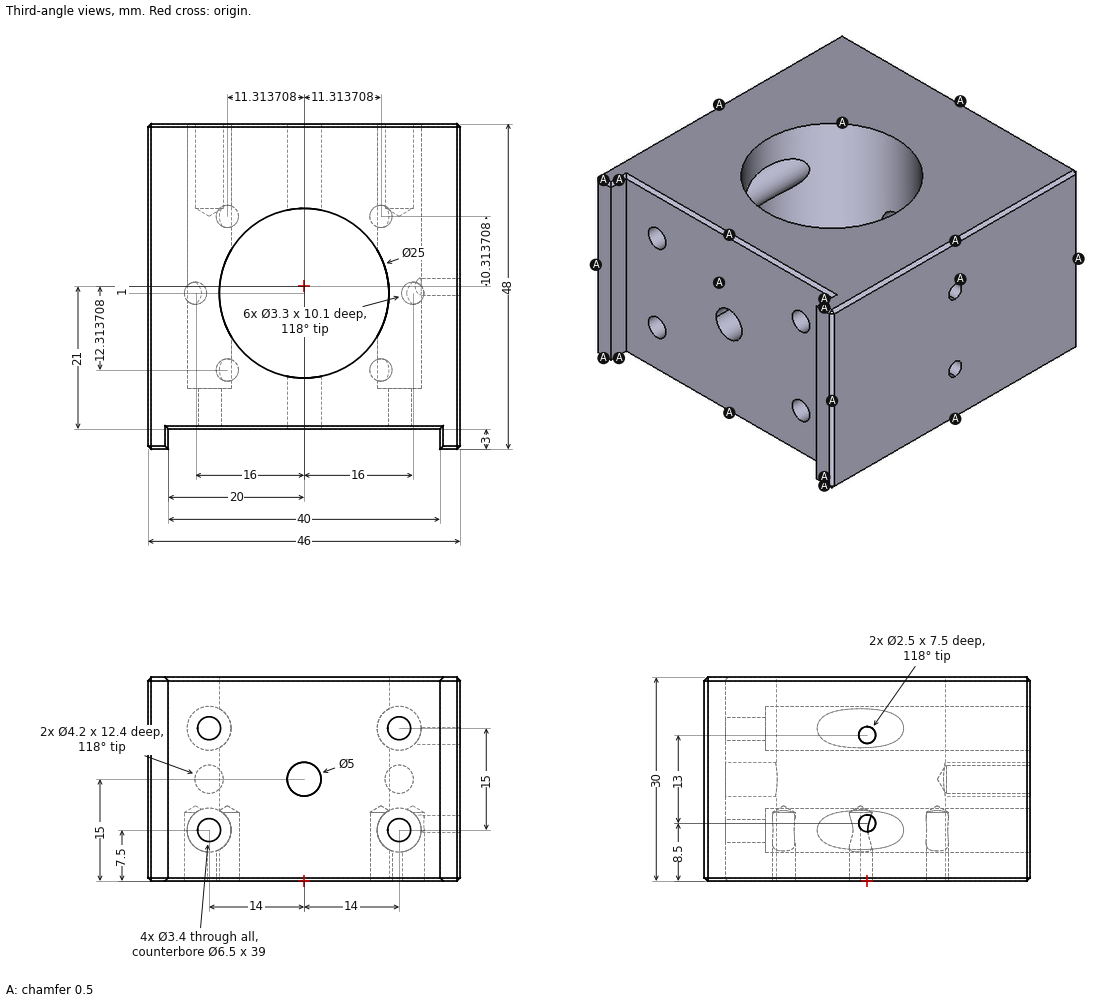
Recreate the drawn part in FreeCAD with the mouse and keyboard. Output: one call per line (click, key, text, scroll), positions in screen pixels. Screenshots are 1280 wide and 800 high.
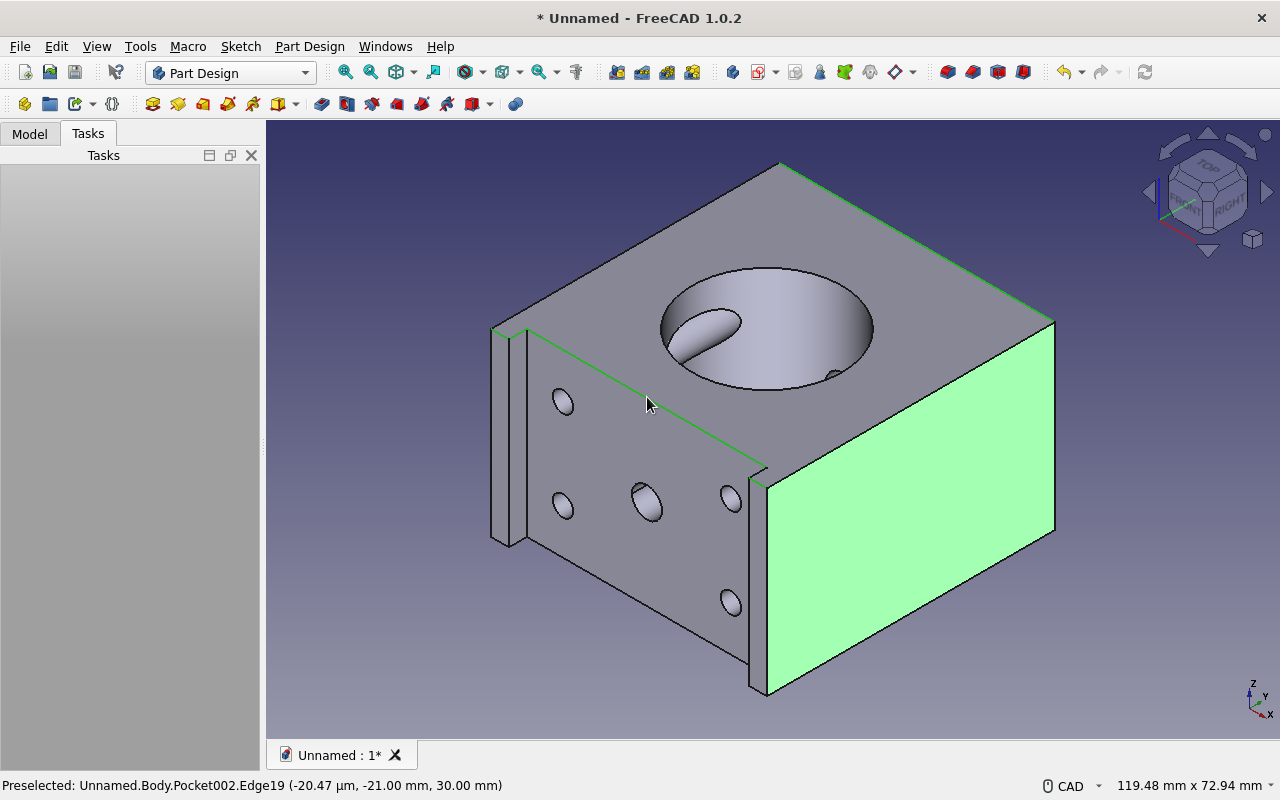
key(2)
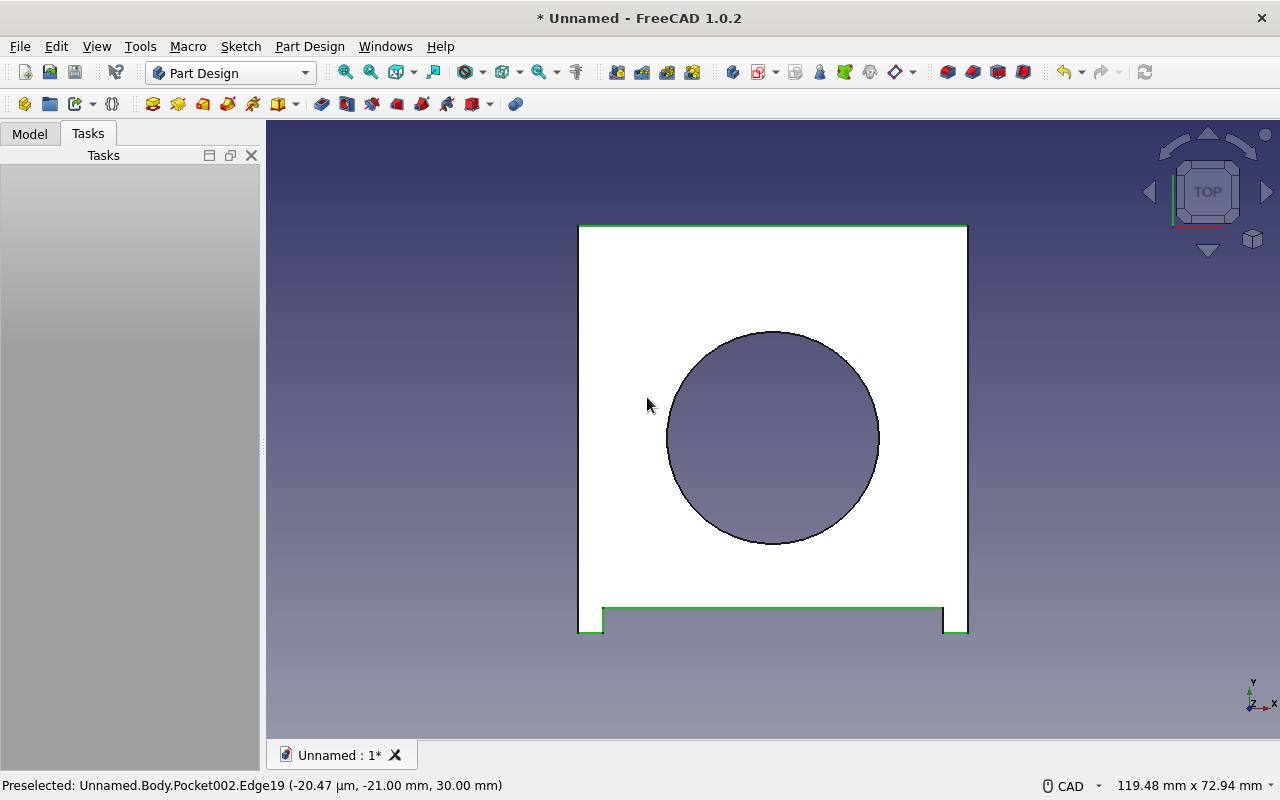
click(943, 619, ctrl)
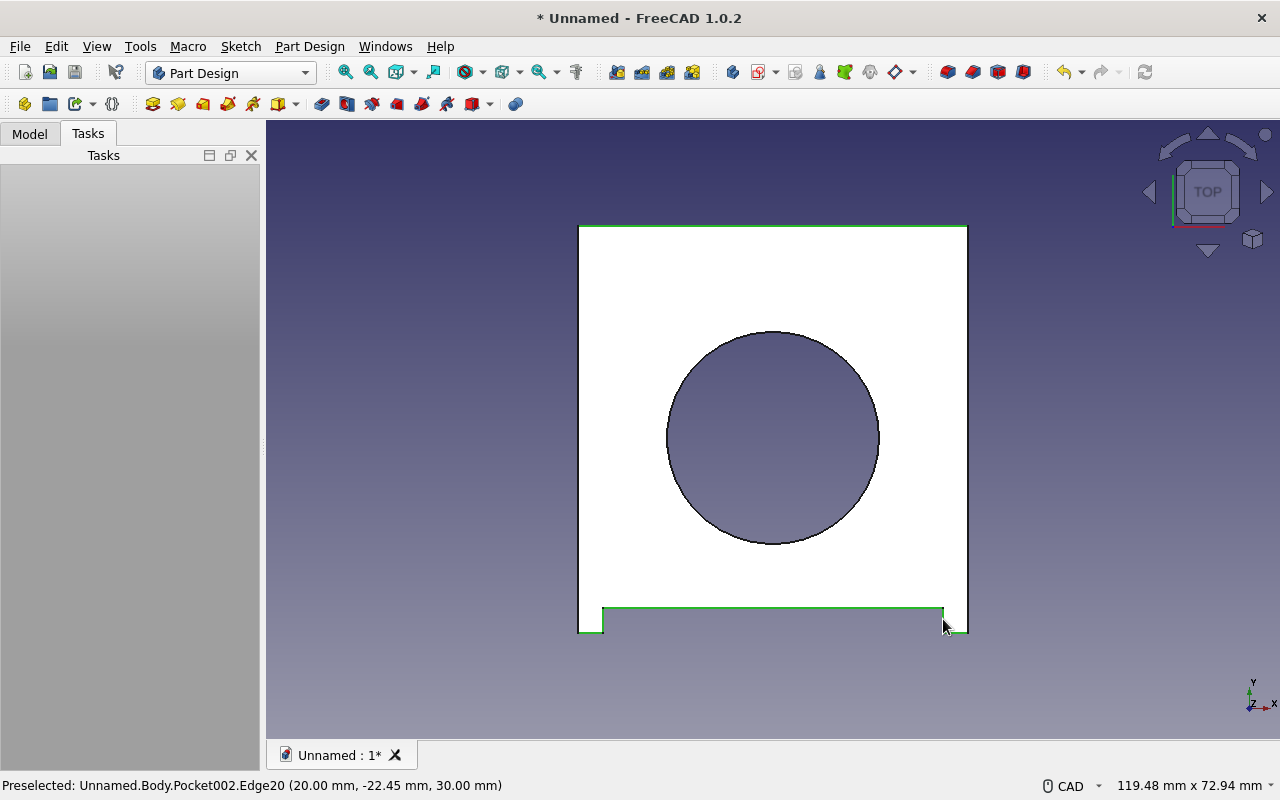
key(1)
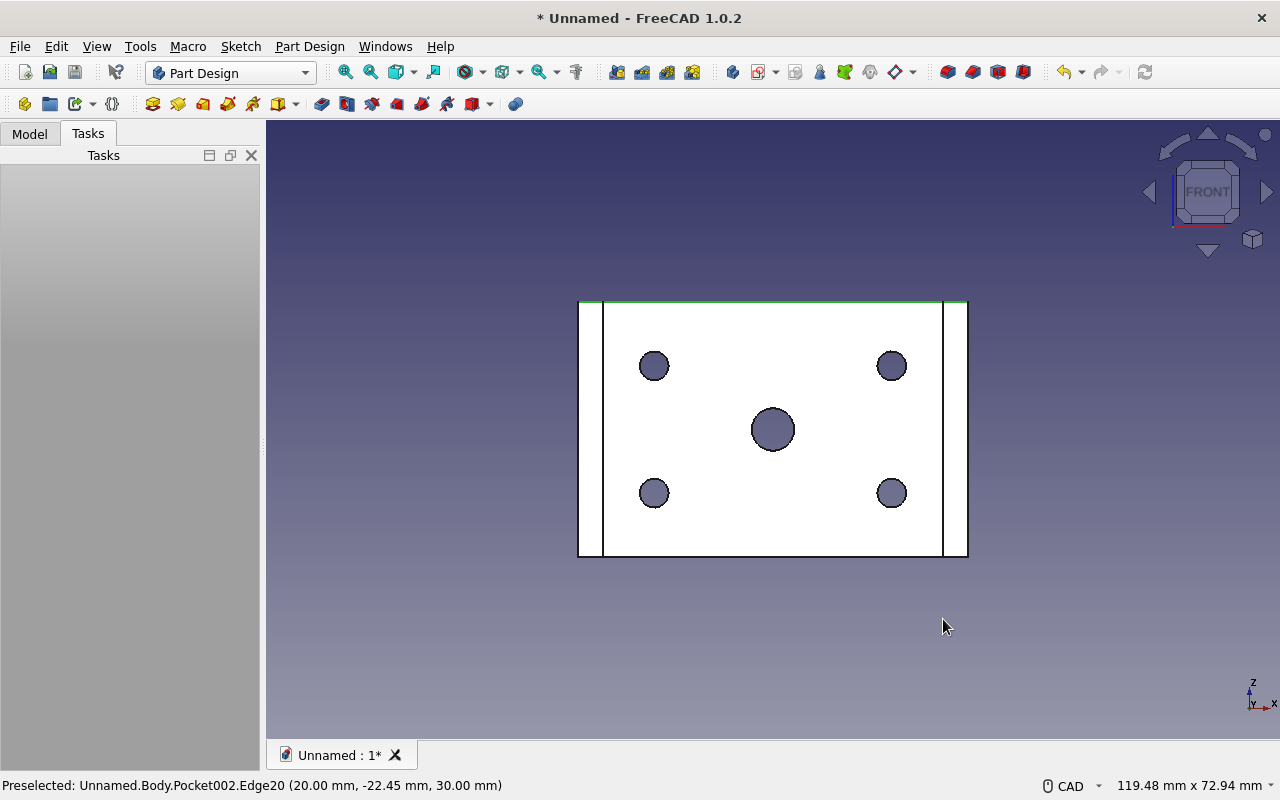
click(346, 72)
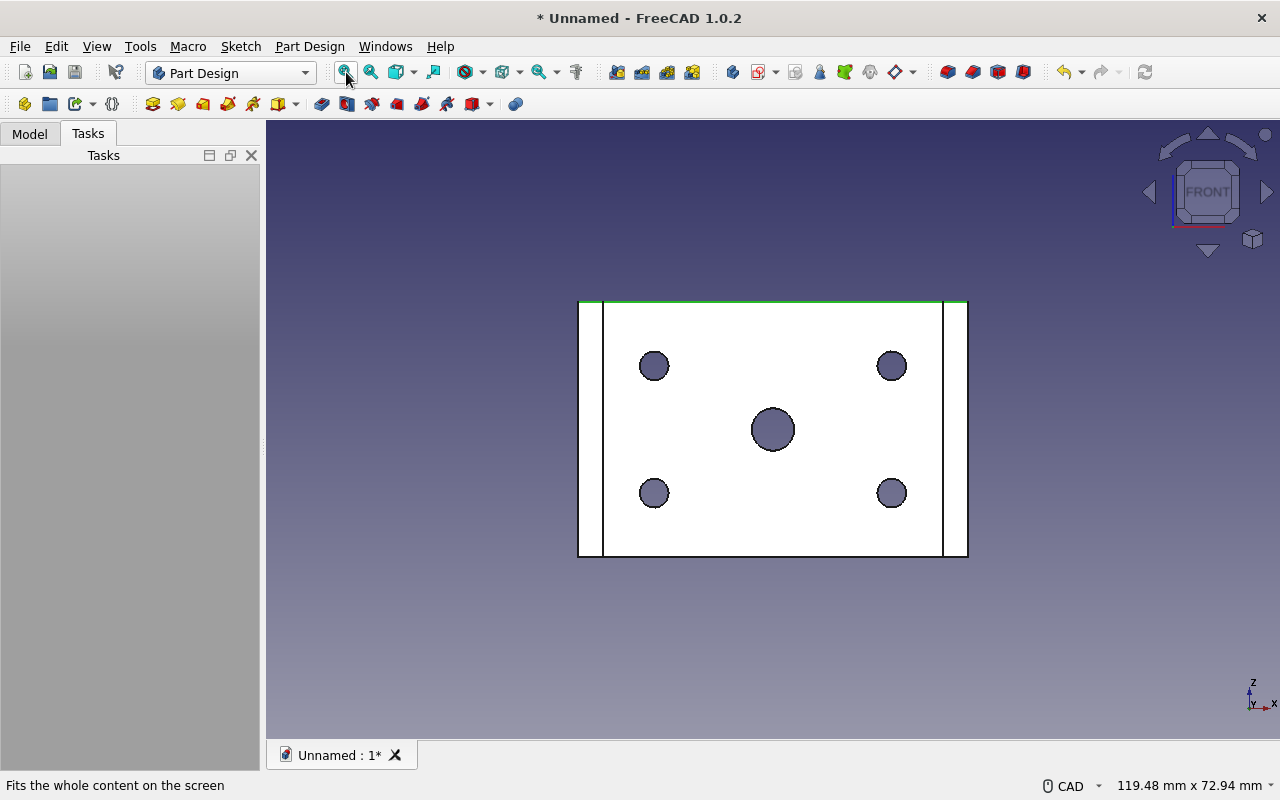
click(955, 556, ctrl)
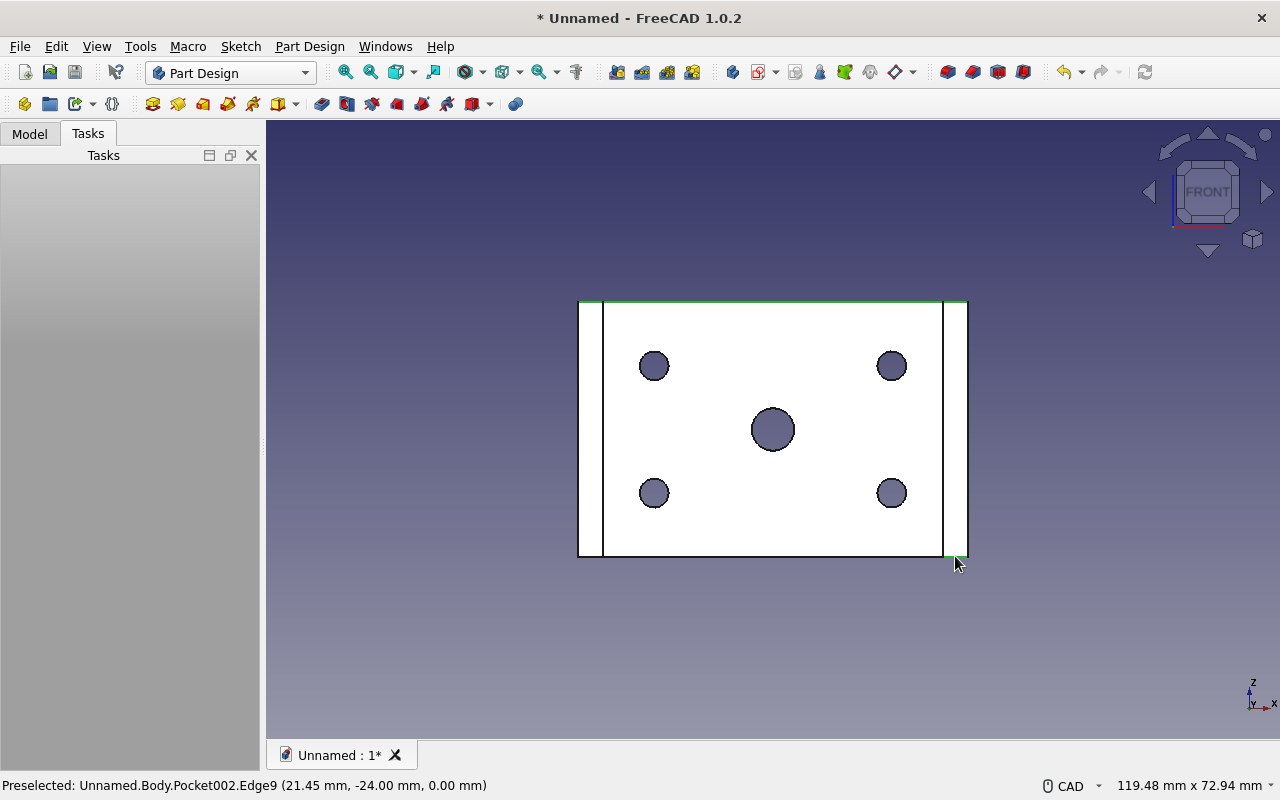
click(773, 556, ctrl)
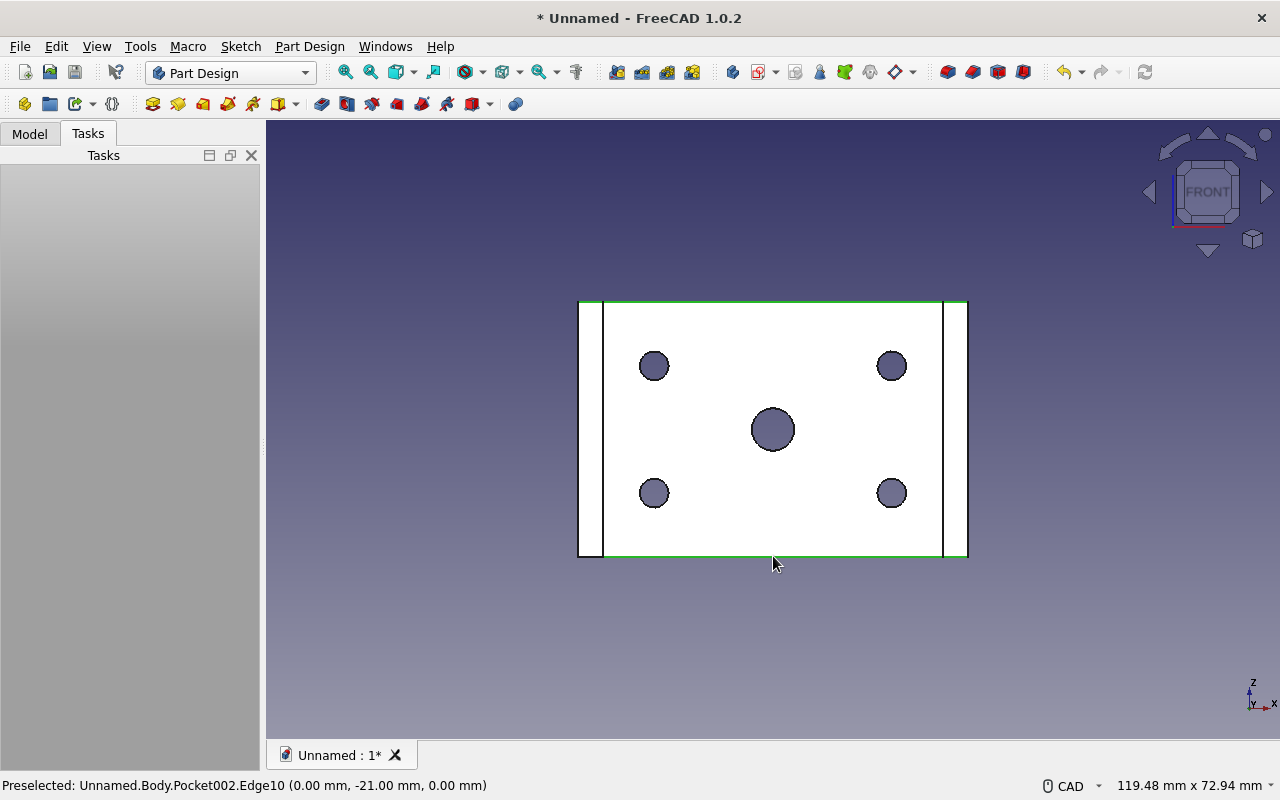
click(591, 556, ctrl)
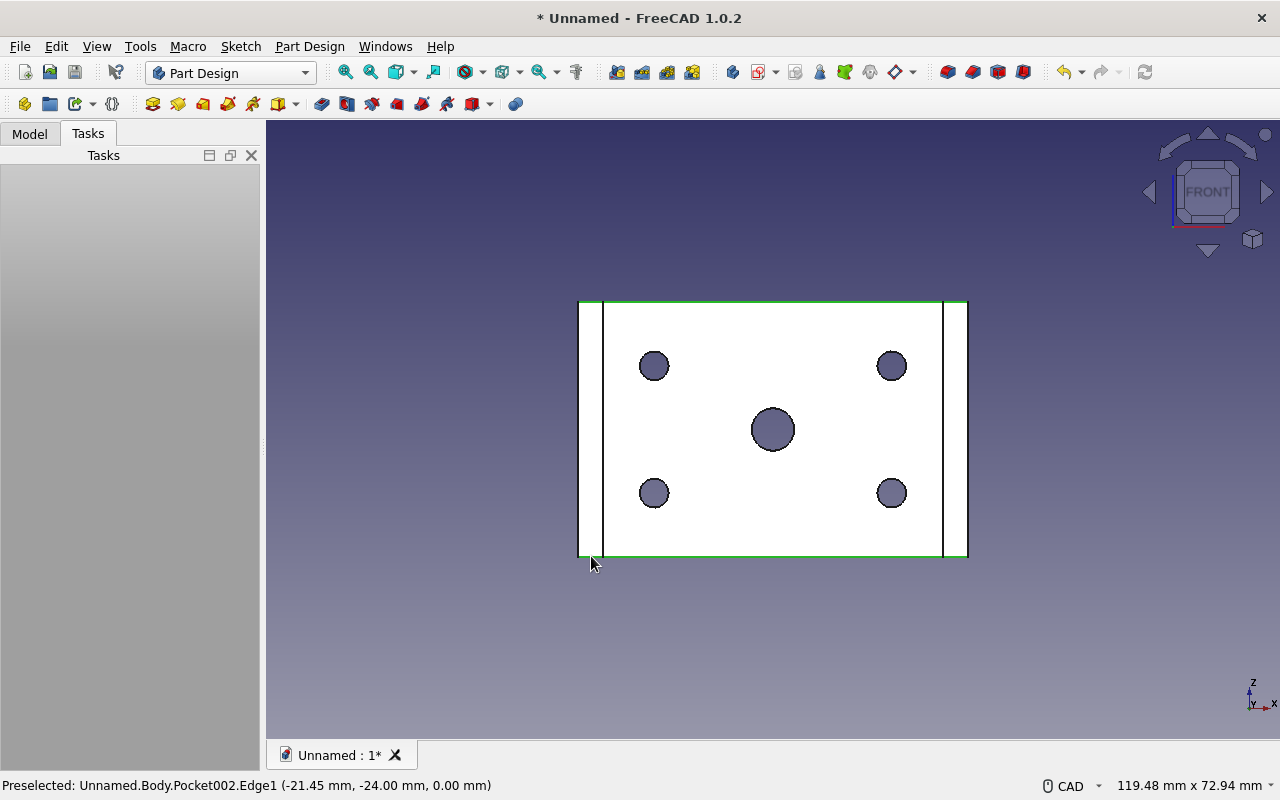
key(3)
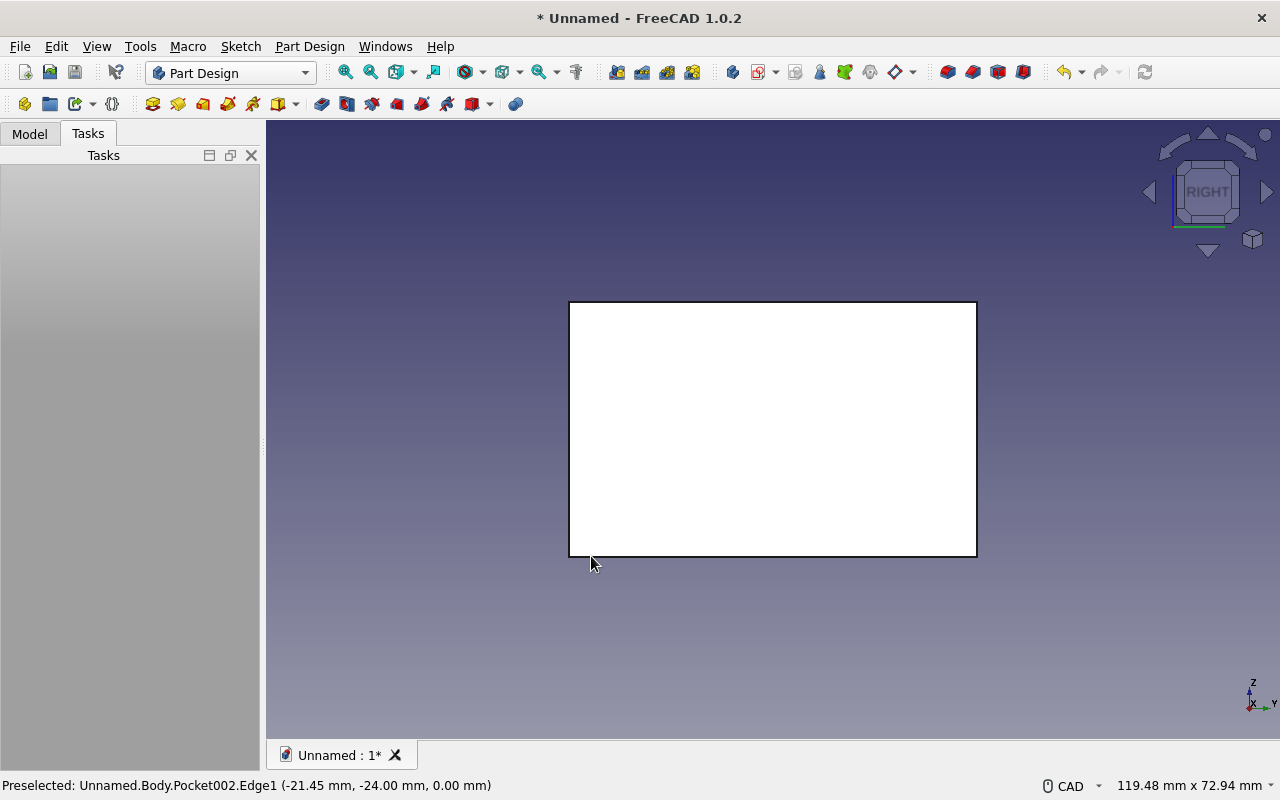
click(346, 72)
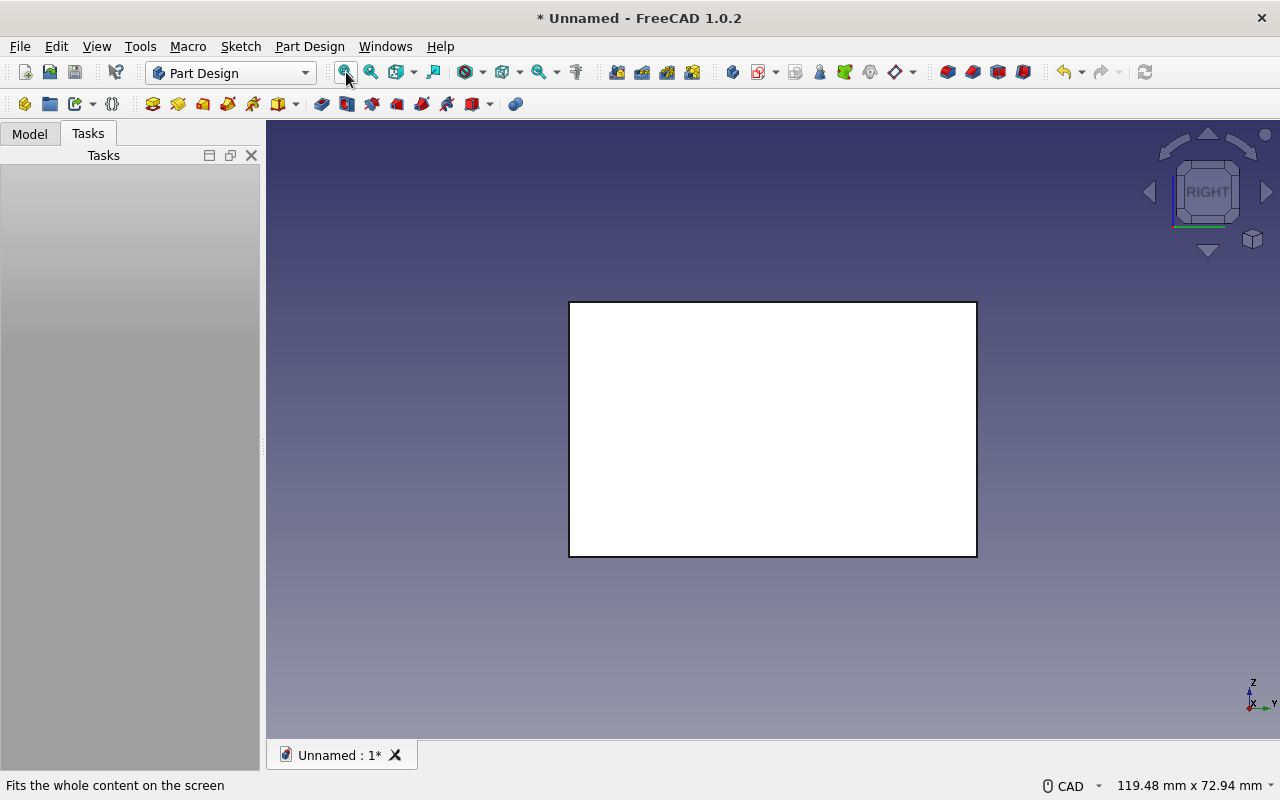
key(5)